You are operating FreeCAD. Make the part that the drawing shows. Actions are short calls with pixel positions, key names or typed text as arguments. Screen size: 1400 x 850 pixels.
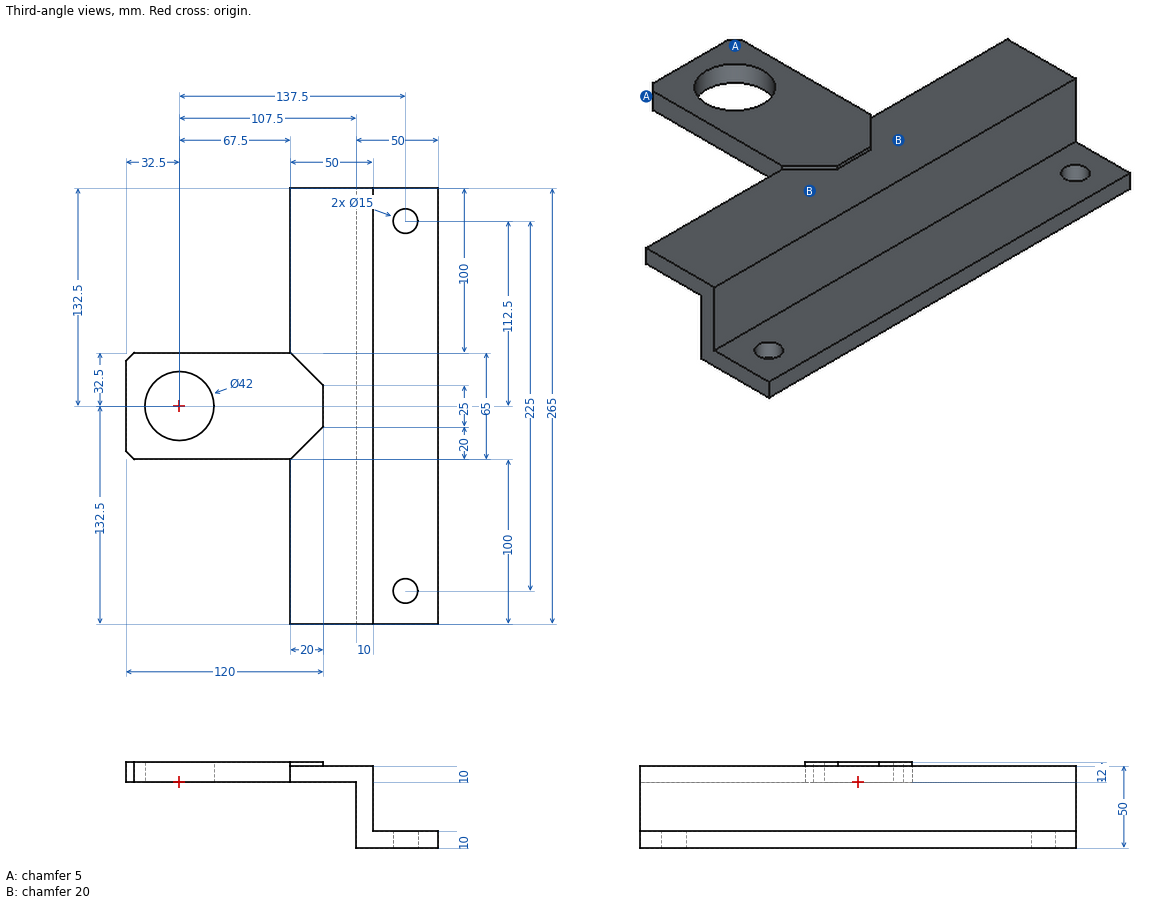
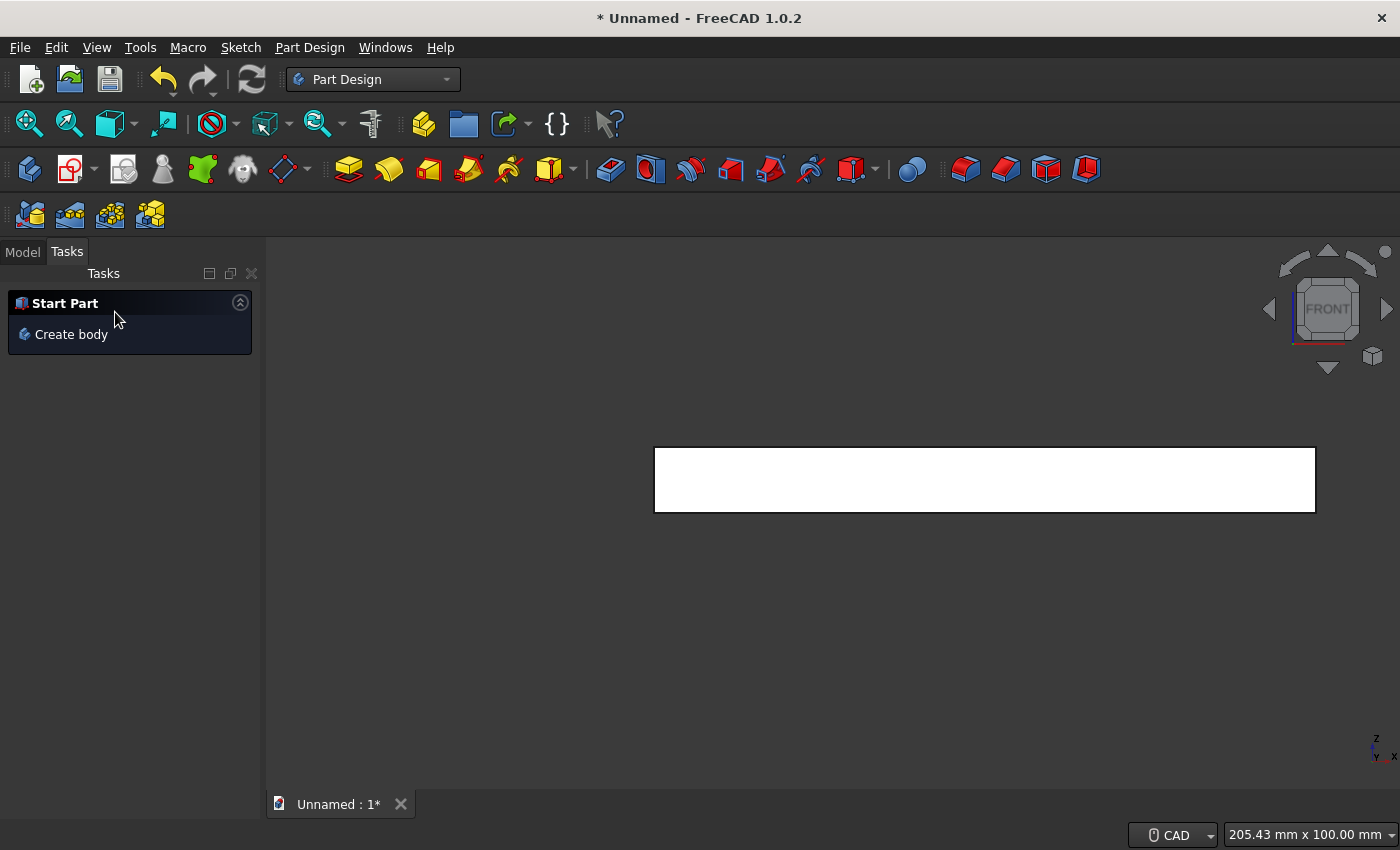
click(654, 479)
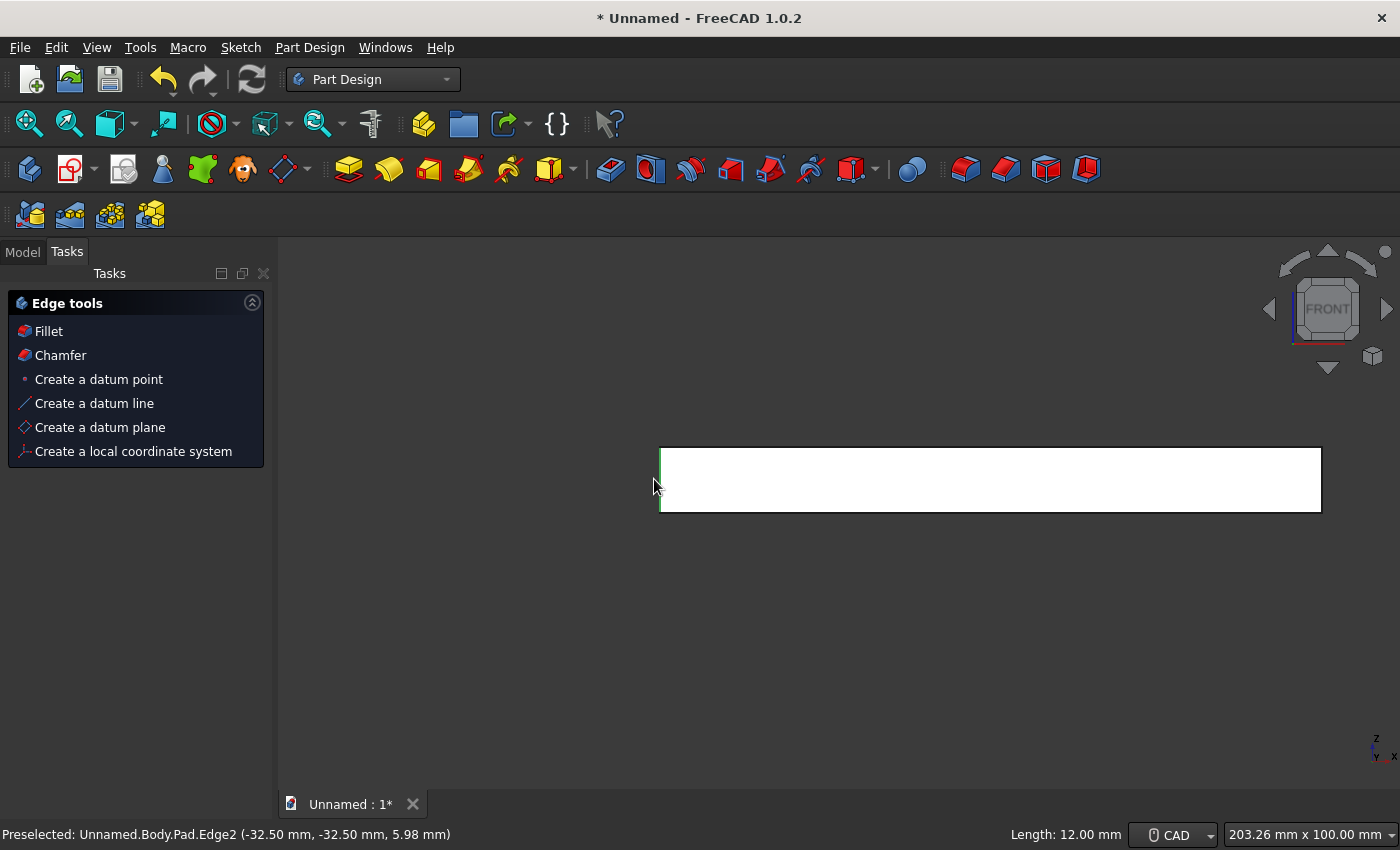
key(3)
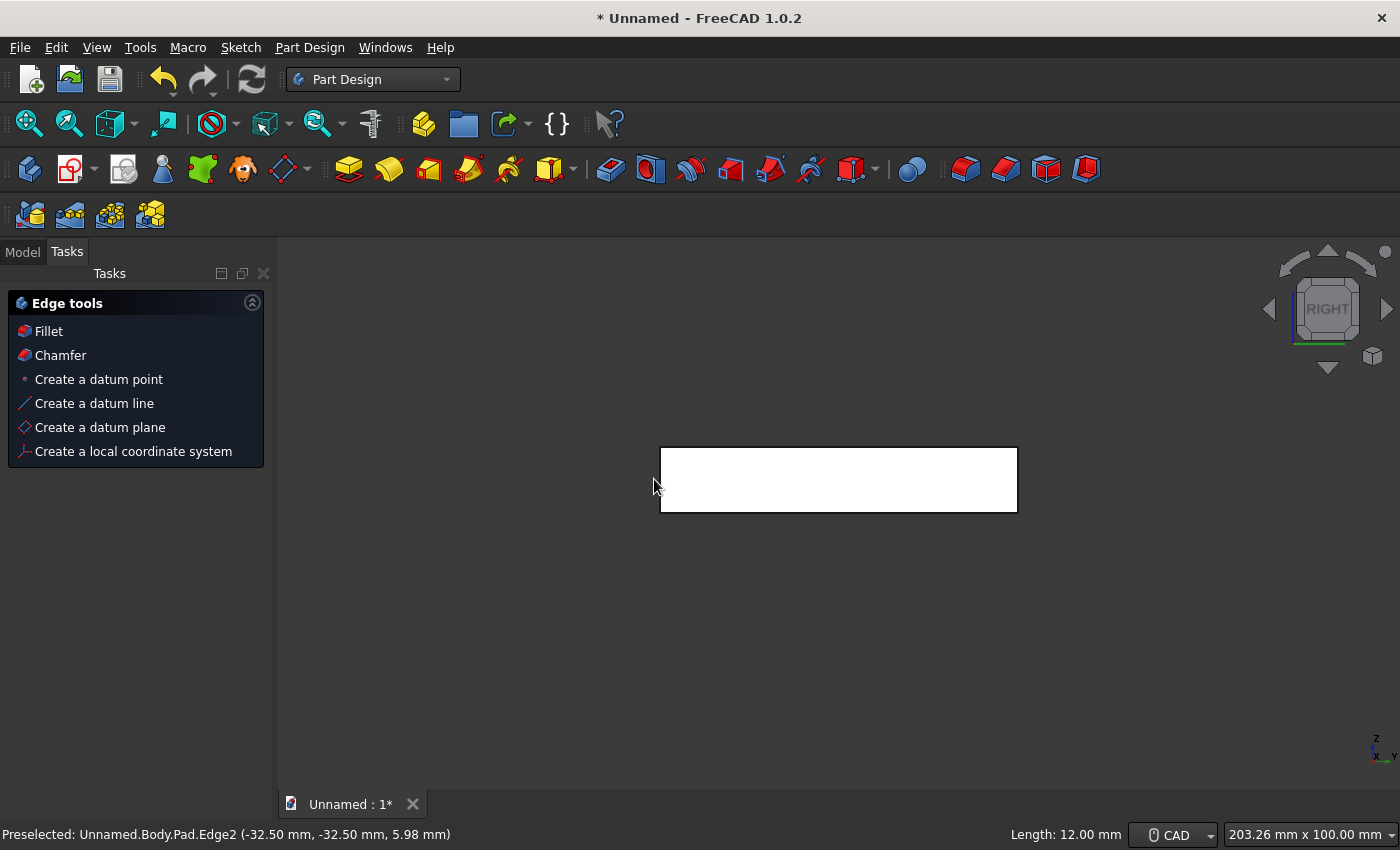
click(30, 124)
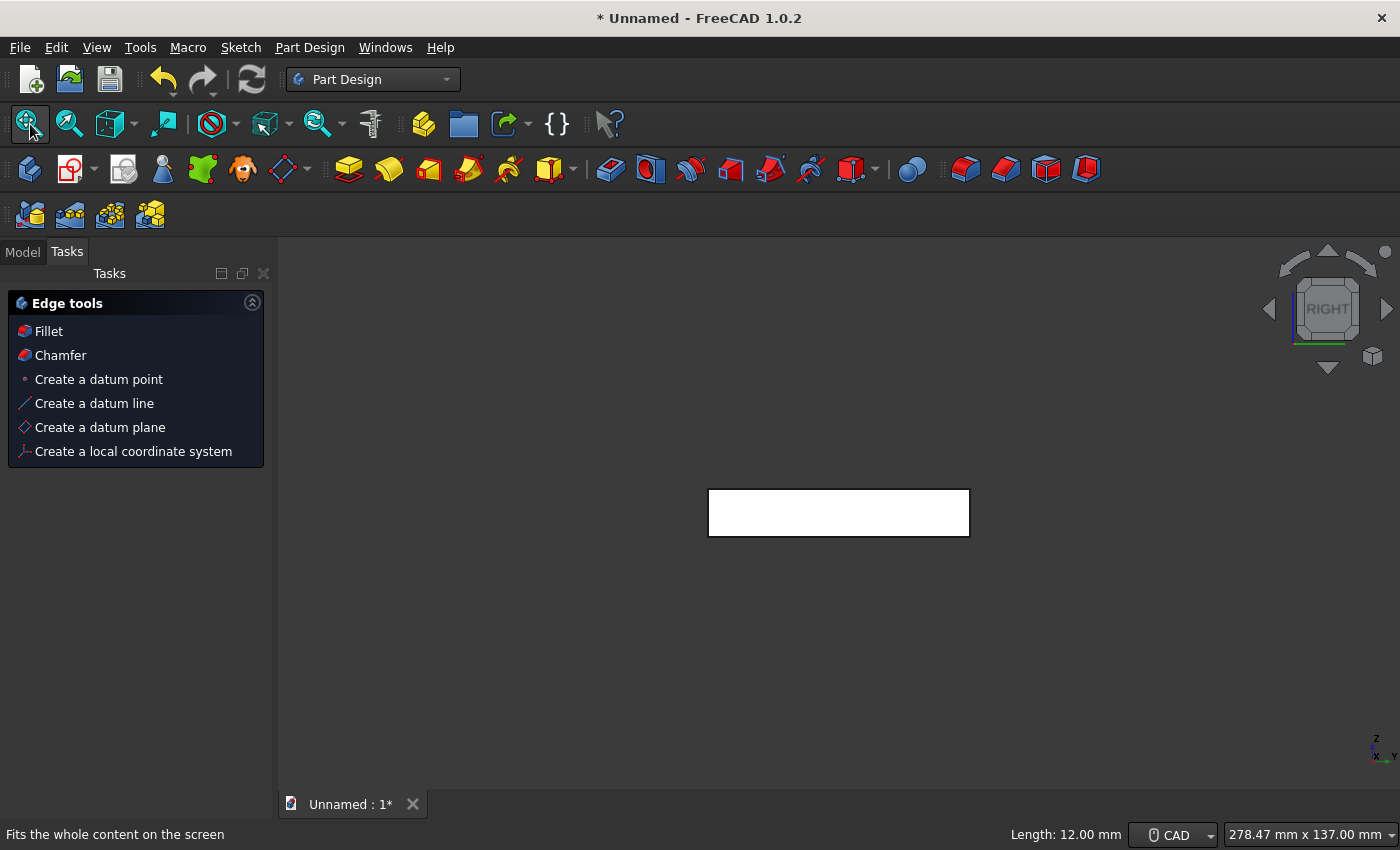
key(5)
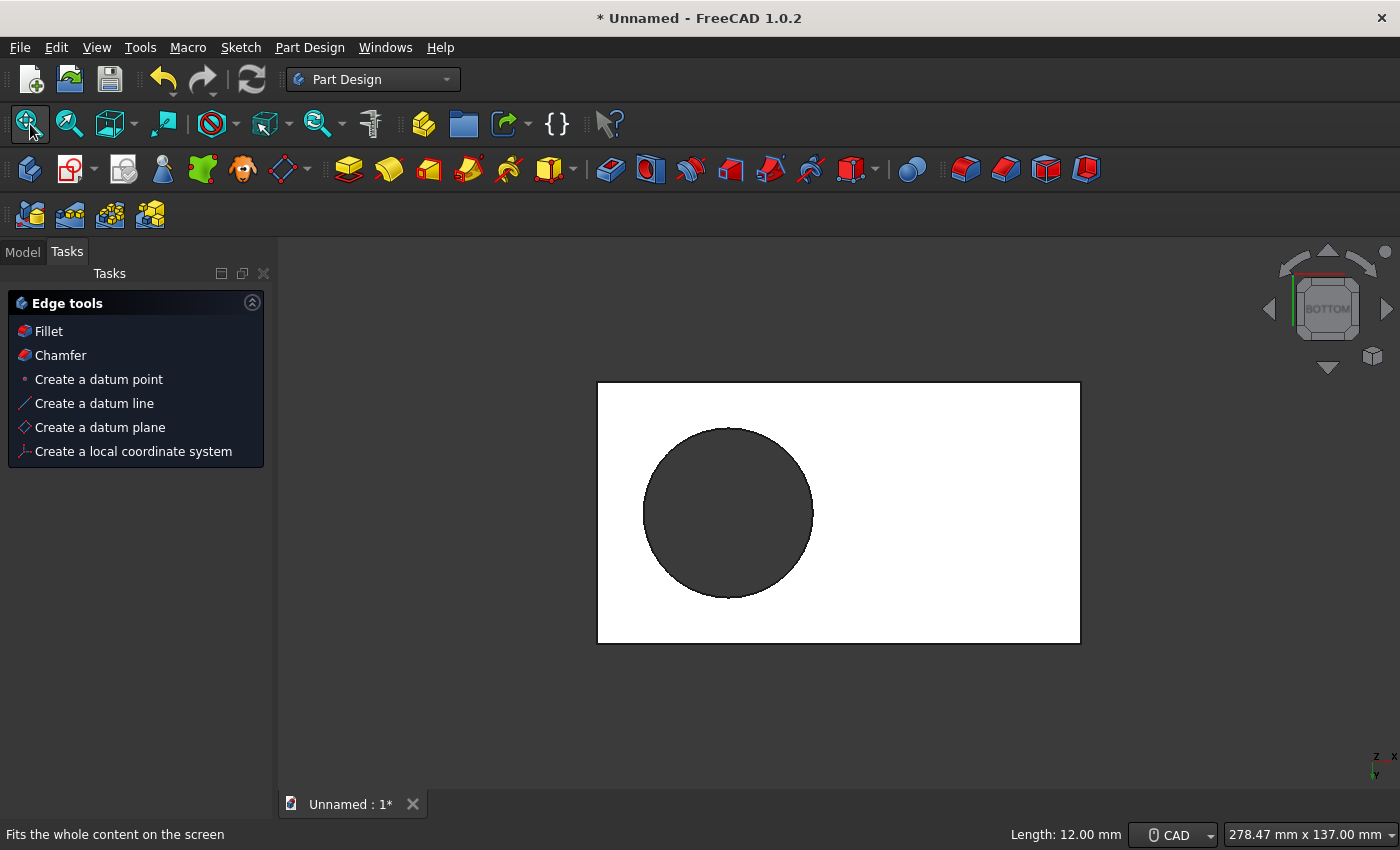
key(4)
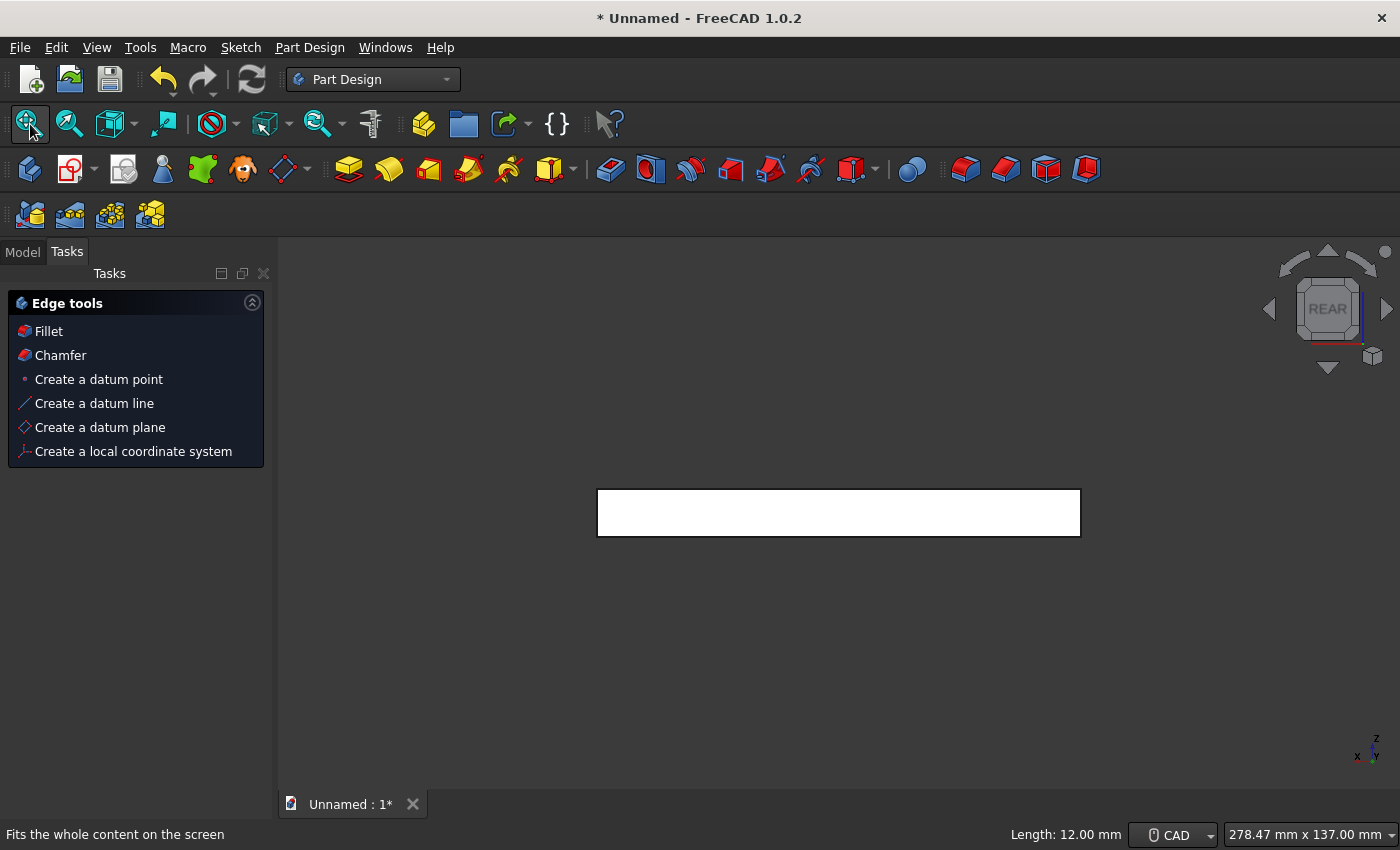
key(v)
key(f)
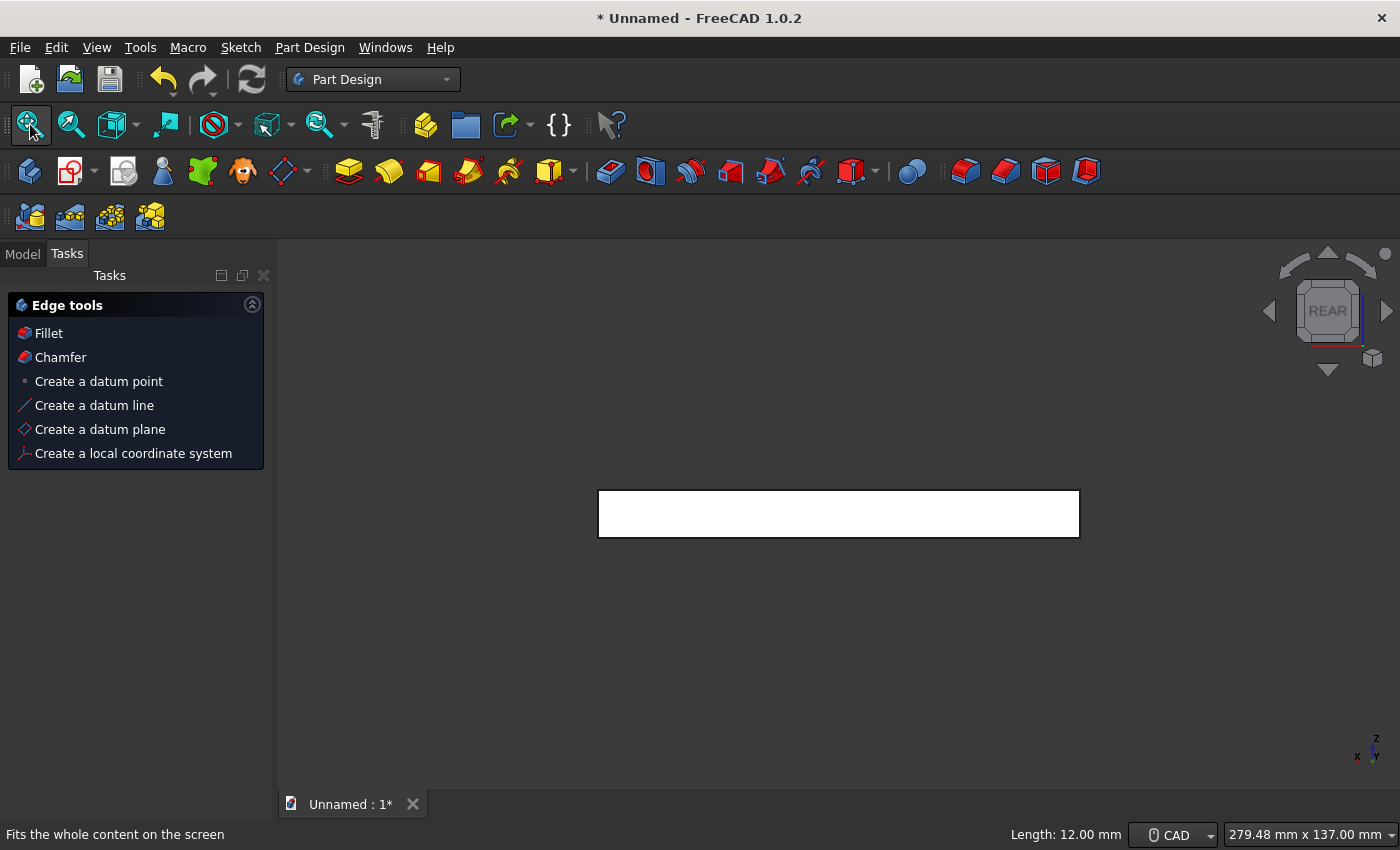
click(1080, 513, ctrl)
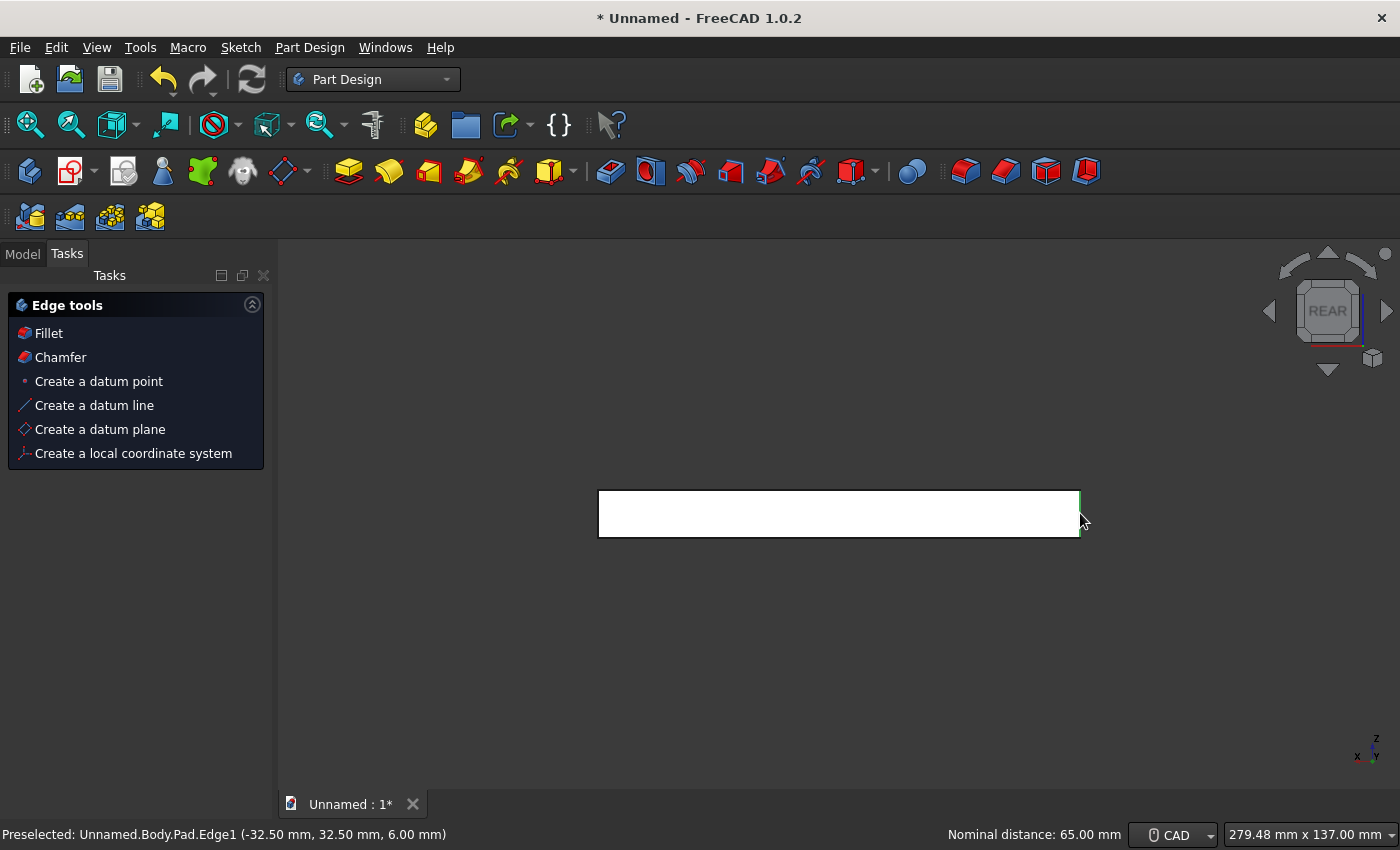
click(1006, 172)